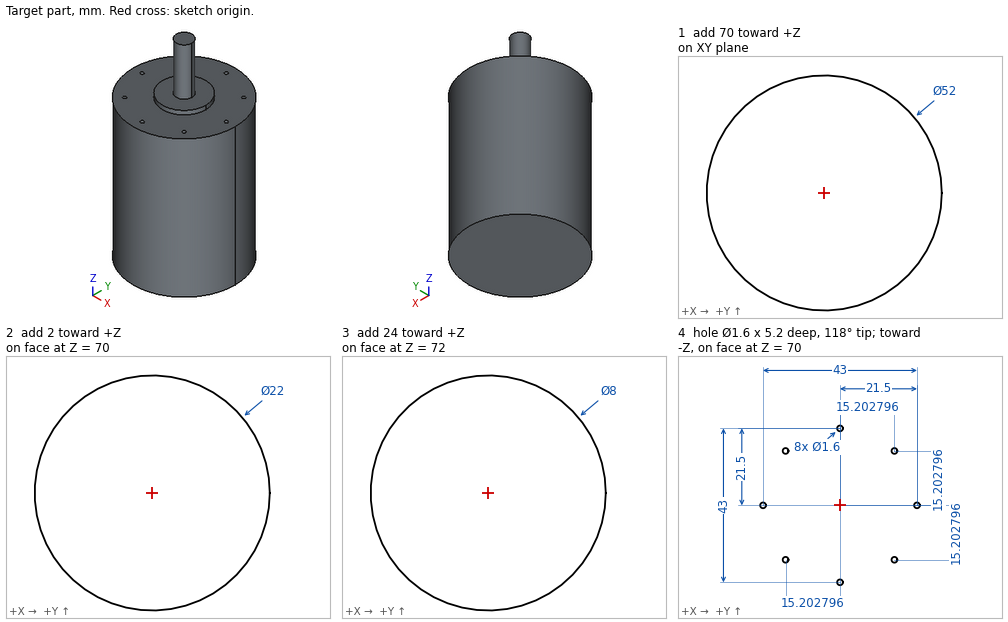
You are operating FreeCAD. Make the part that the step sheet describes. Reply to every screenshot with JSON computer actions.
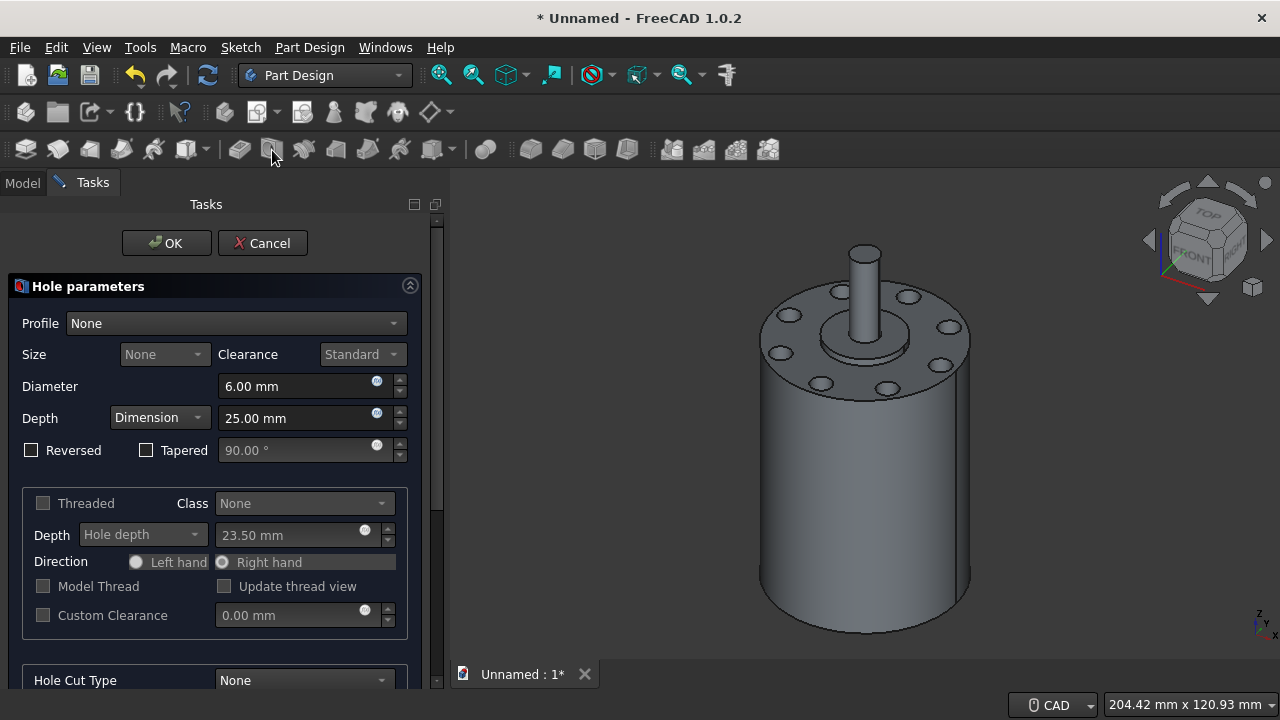
{"action": "triple_click", "coordinate": [305, 386]}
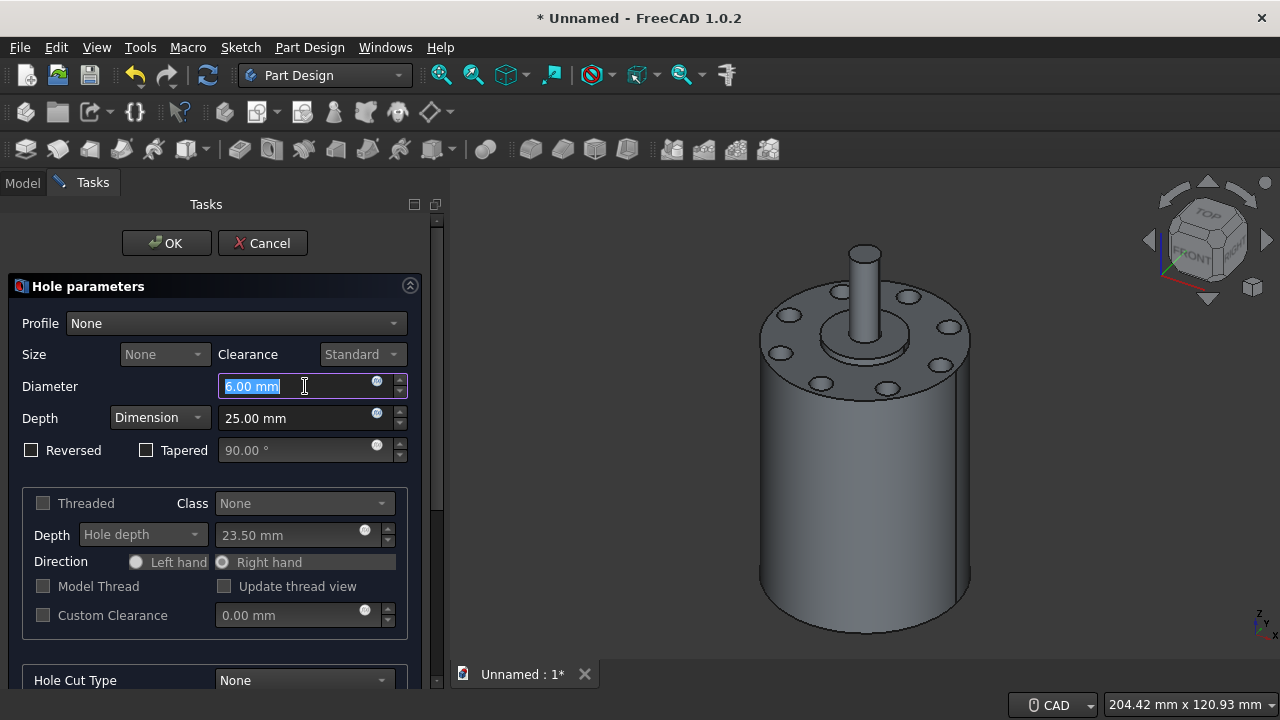
{"action": "type", "text": "1.6"}
{"action": "key", "text": "Tab"}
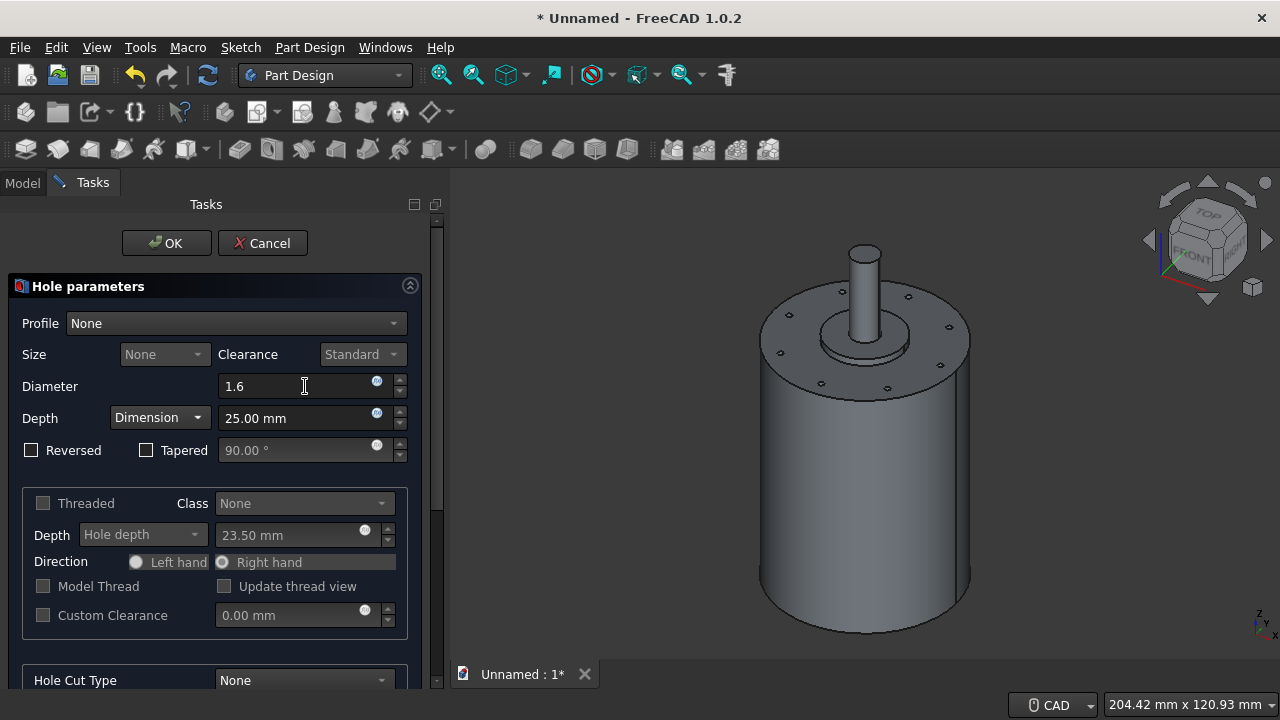
{"action": "triple_click", "coordinate": [305, 418]}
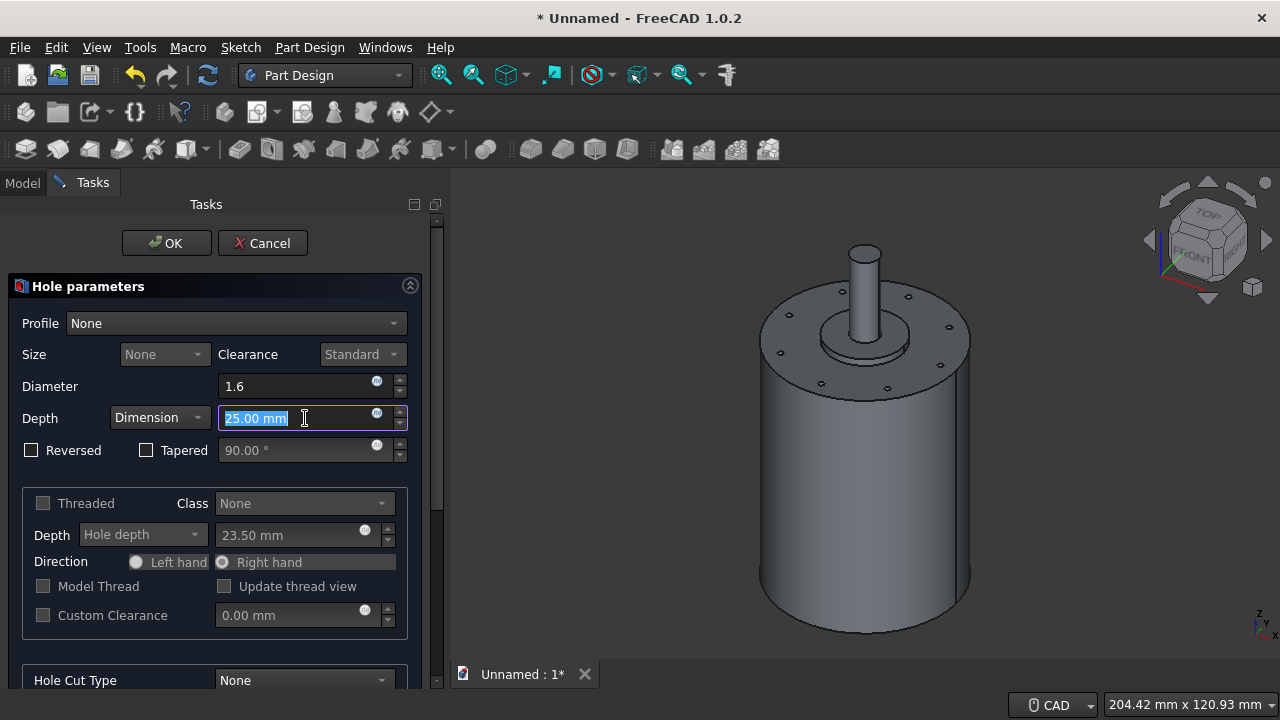
{"action": "type", "text": "5.2"}
{"action": "key", "text": "Tab"}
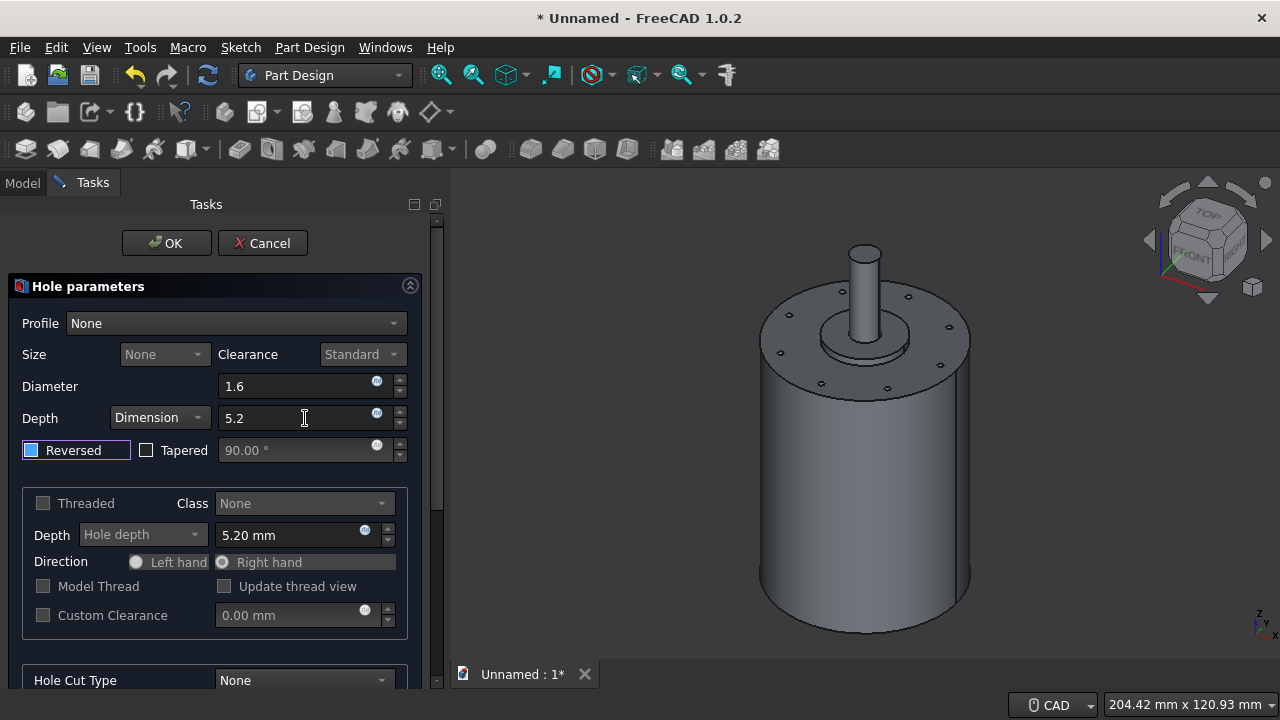
{"action": "left_click", "coordinate": [167, 243]}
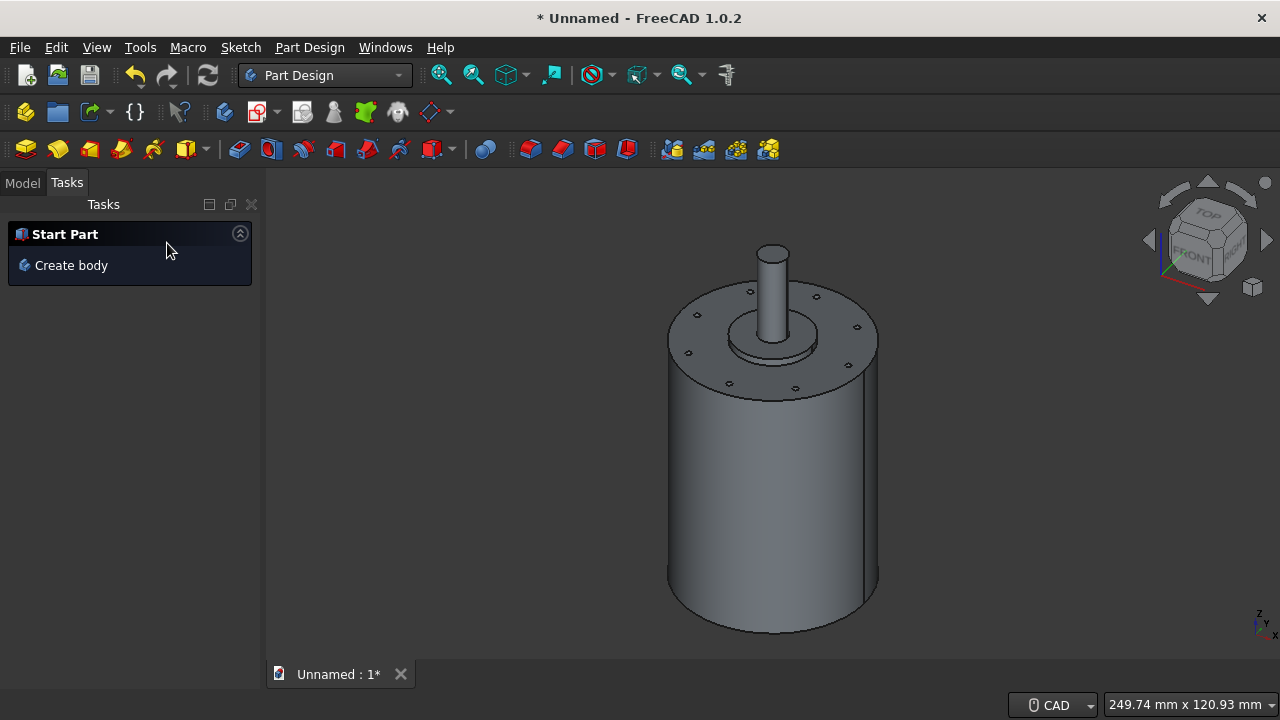
{"action": "key", "text": "0"}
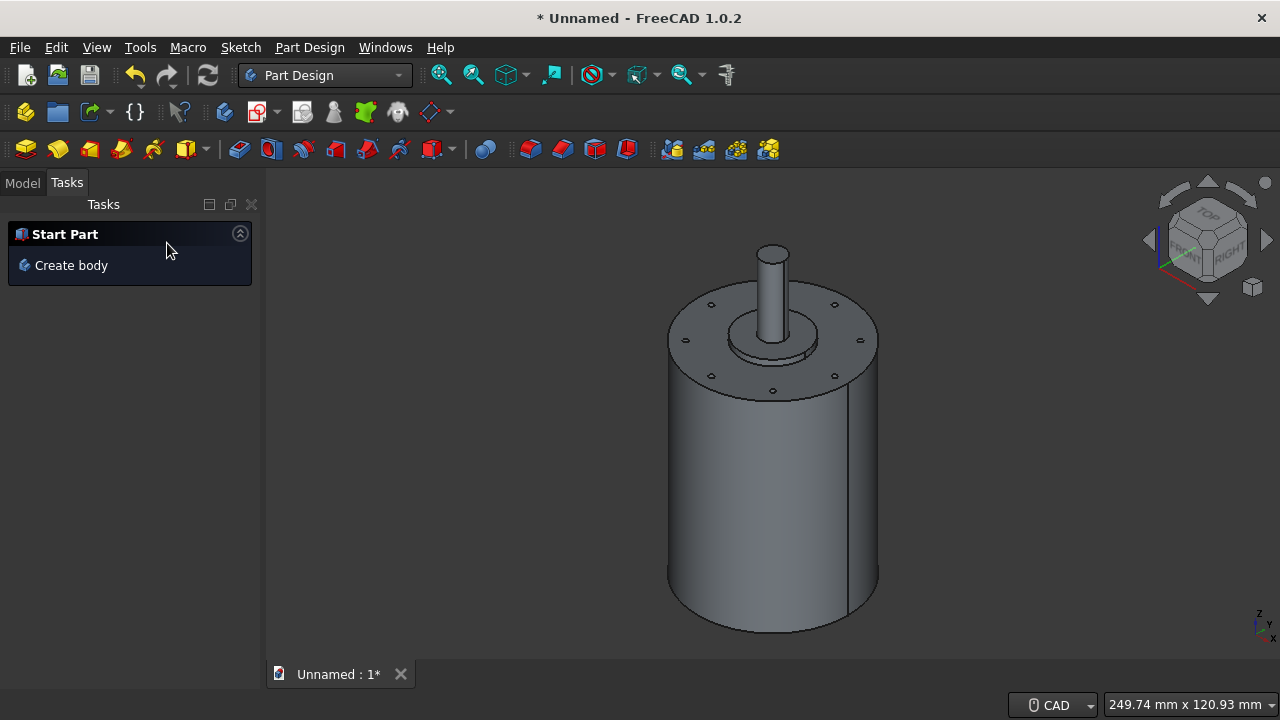
{"action": "left_click", "coordinate": [442, 76]}